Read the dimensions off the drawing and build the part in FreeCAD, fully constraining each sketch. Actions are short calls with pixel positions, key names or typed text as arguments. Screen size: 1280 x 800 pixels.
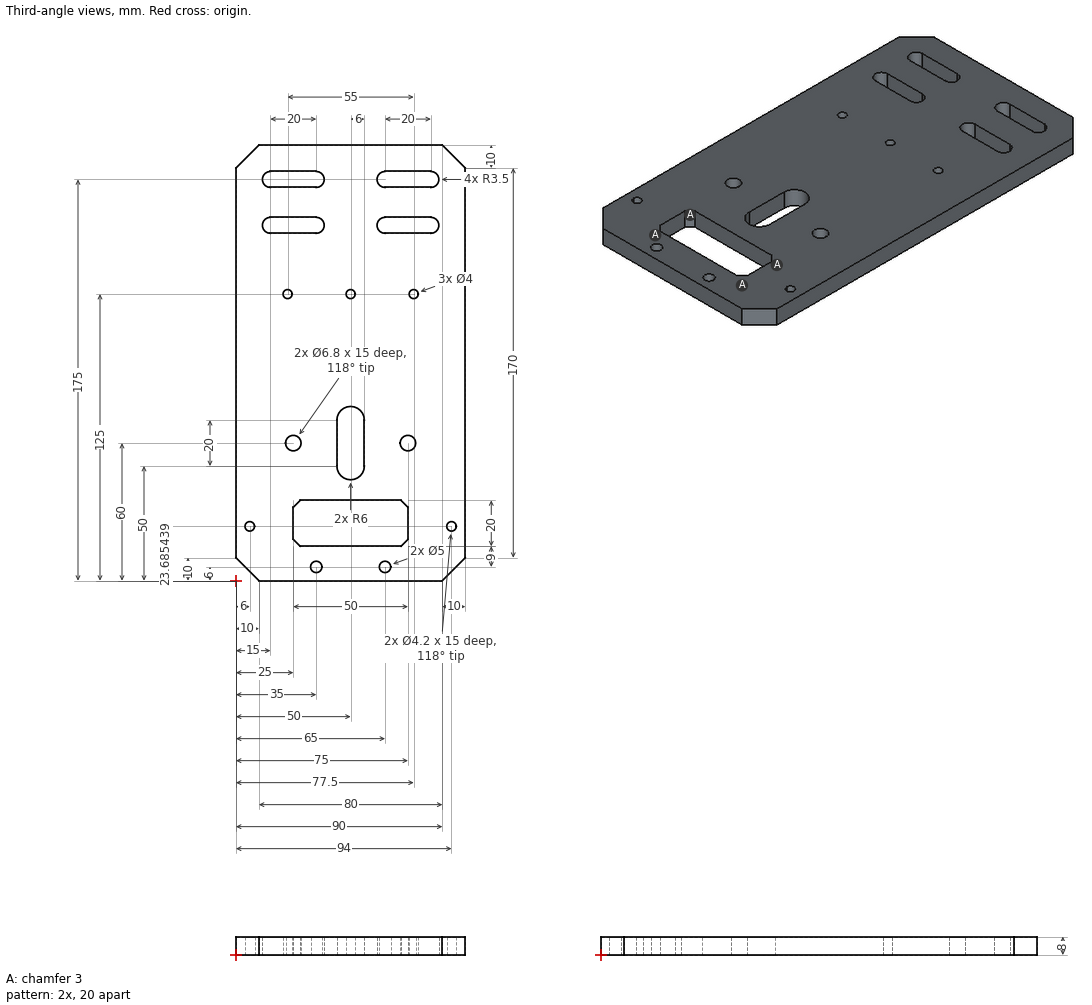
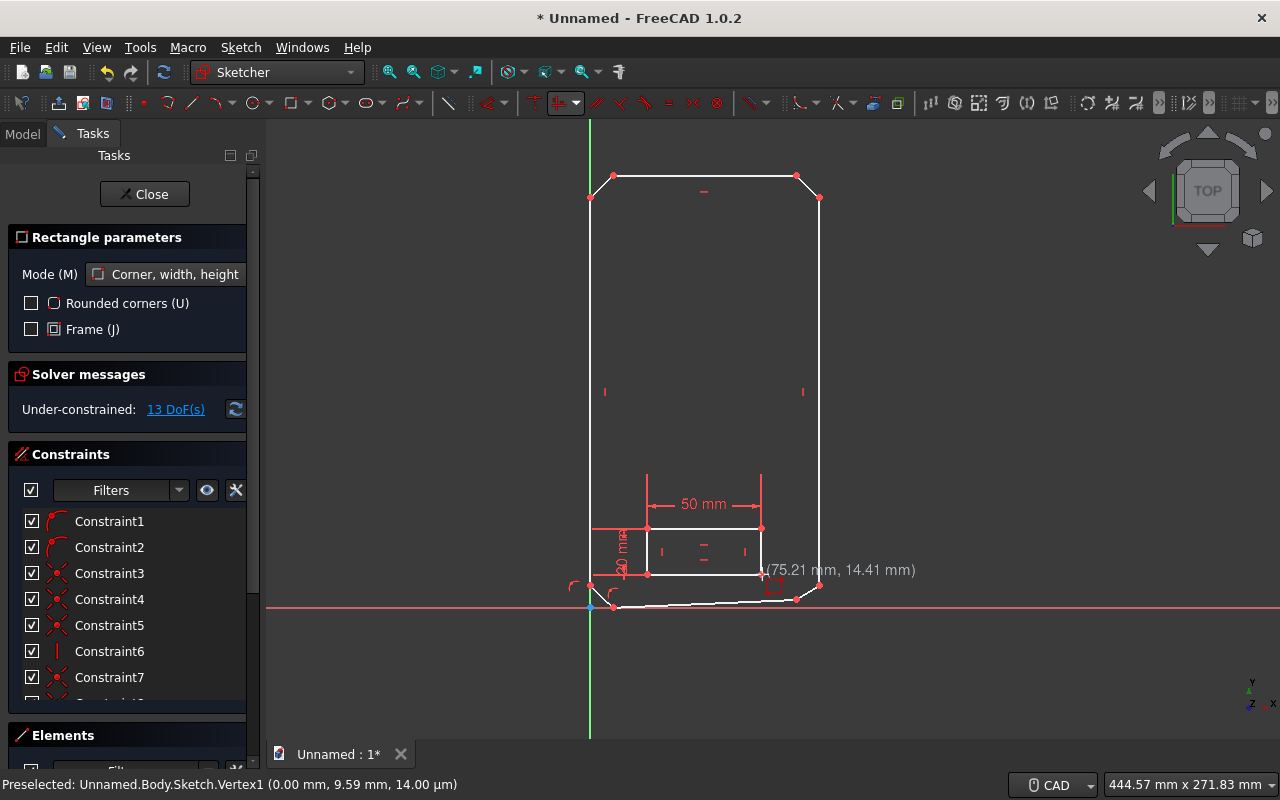
click(366, 104)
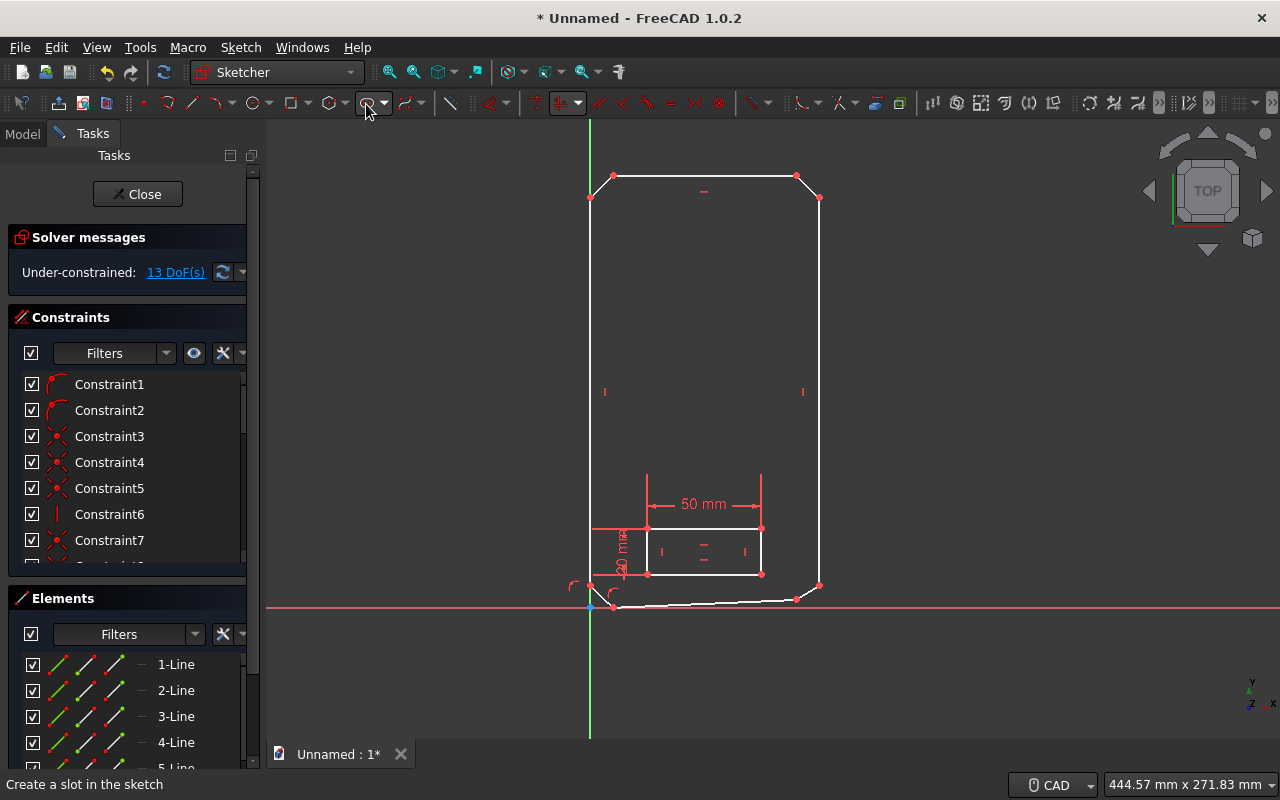
scroll(704, 494, up, 3)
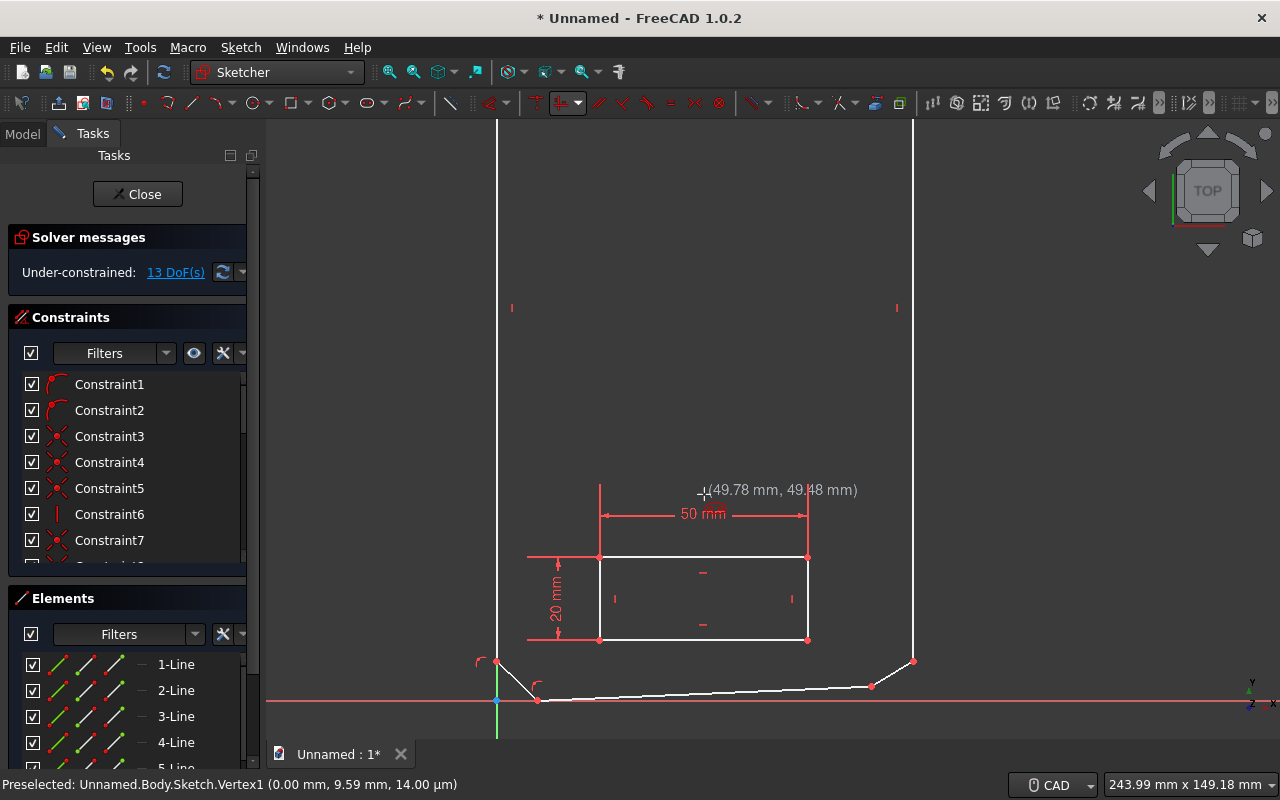
click(705, 493)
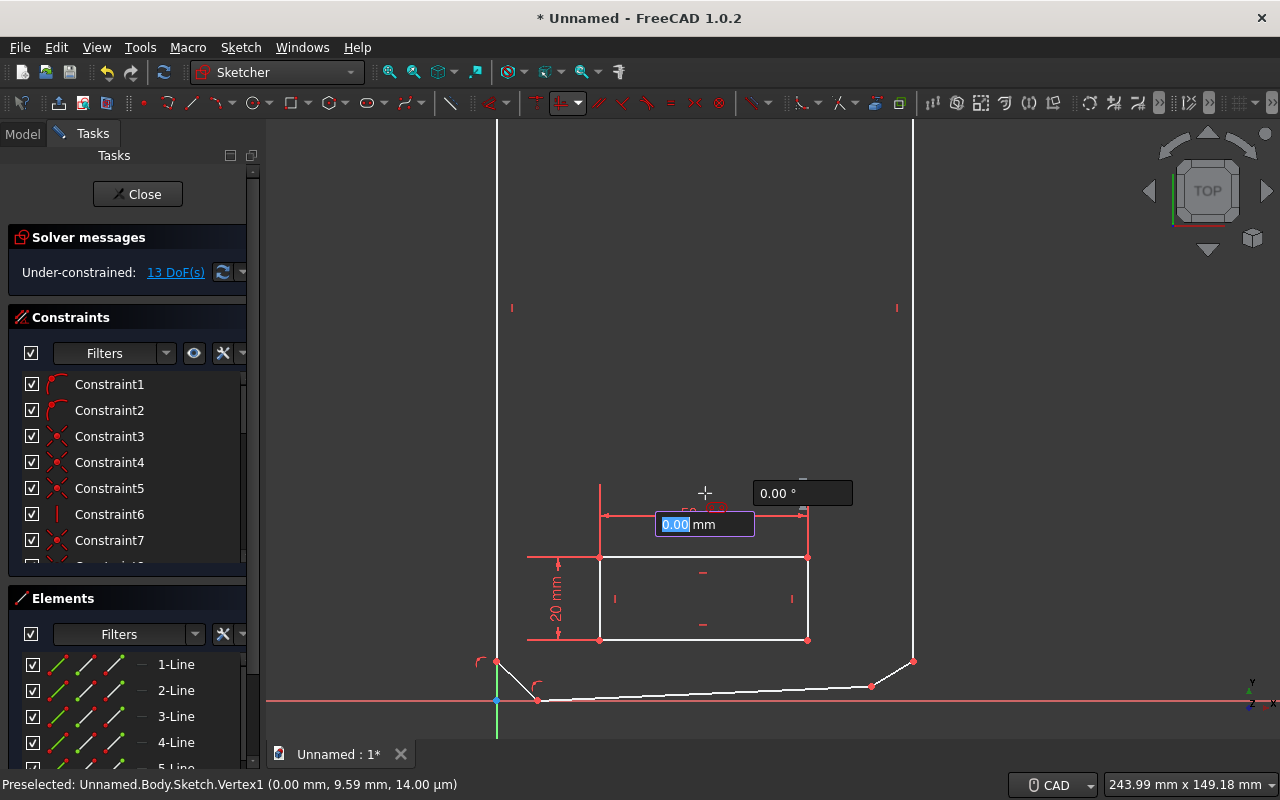
click(705, 410)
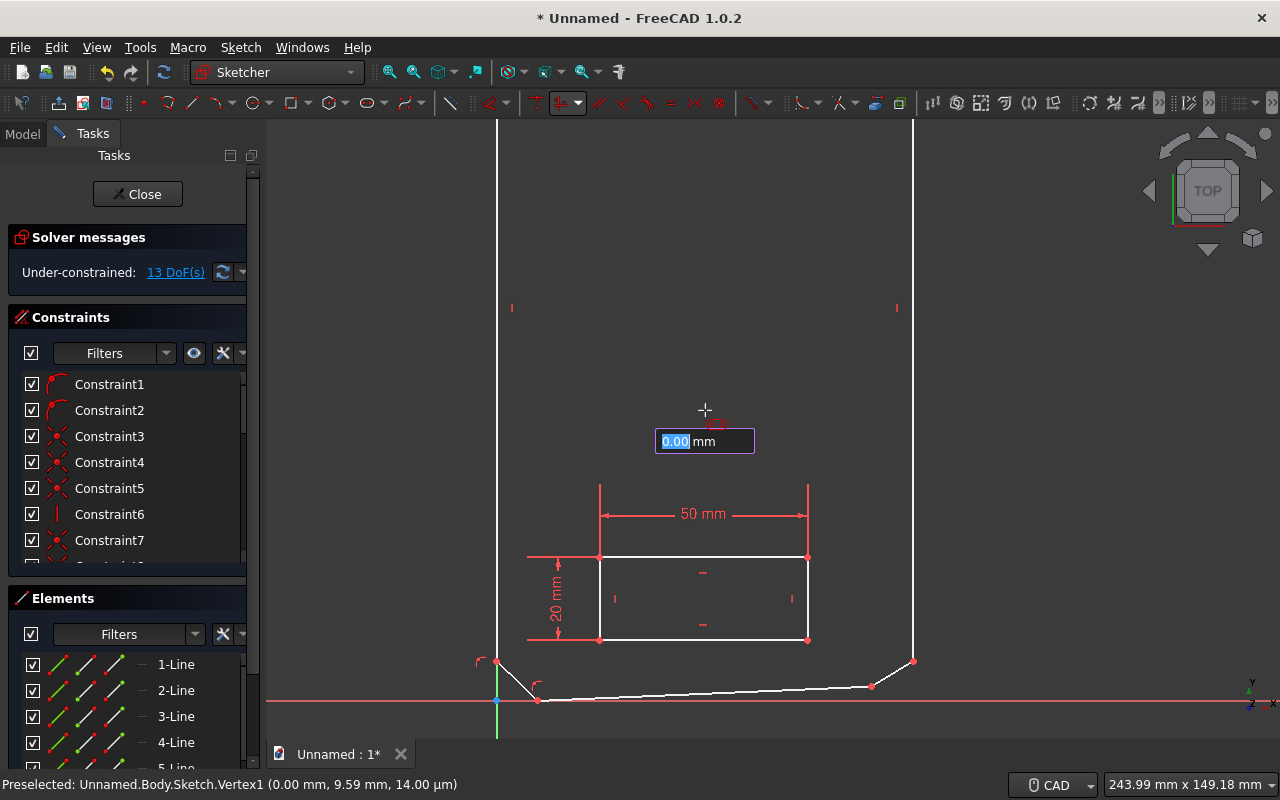
click(729, 452)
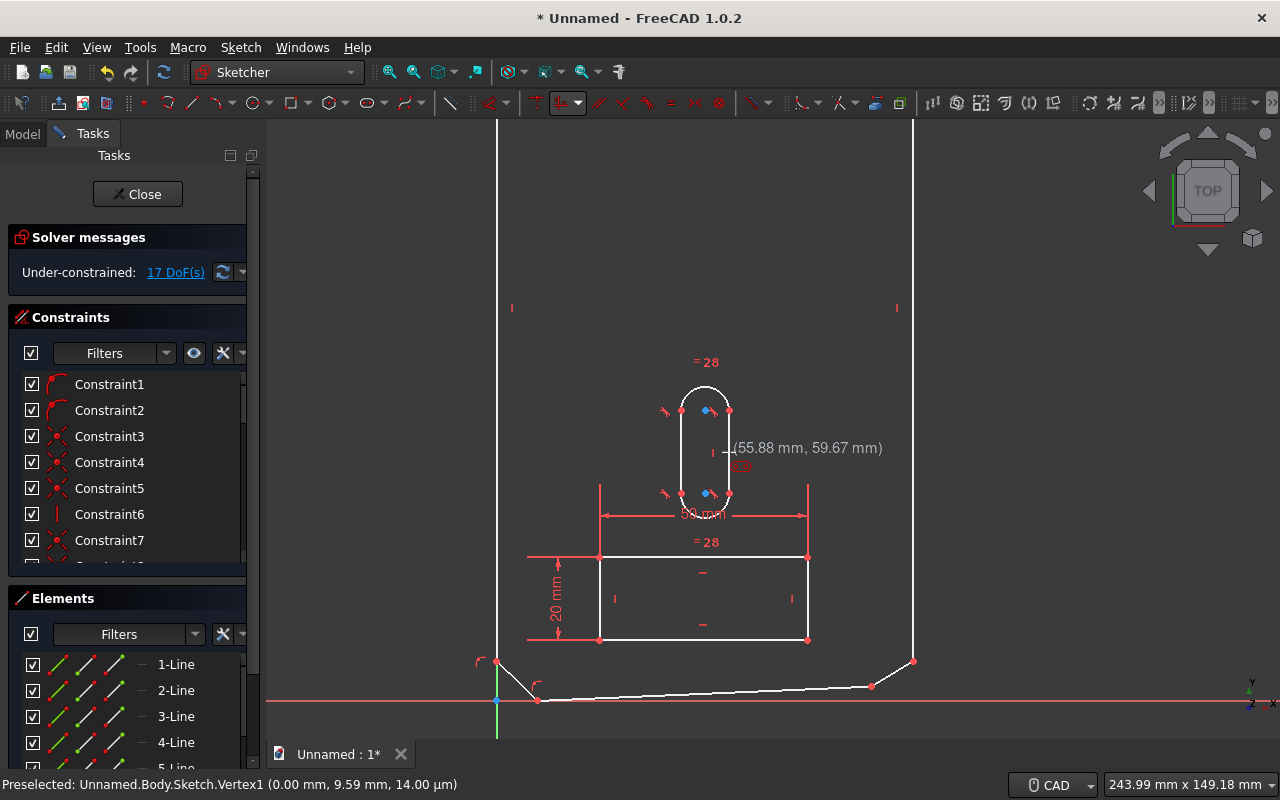
click(254, 104)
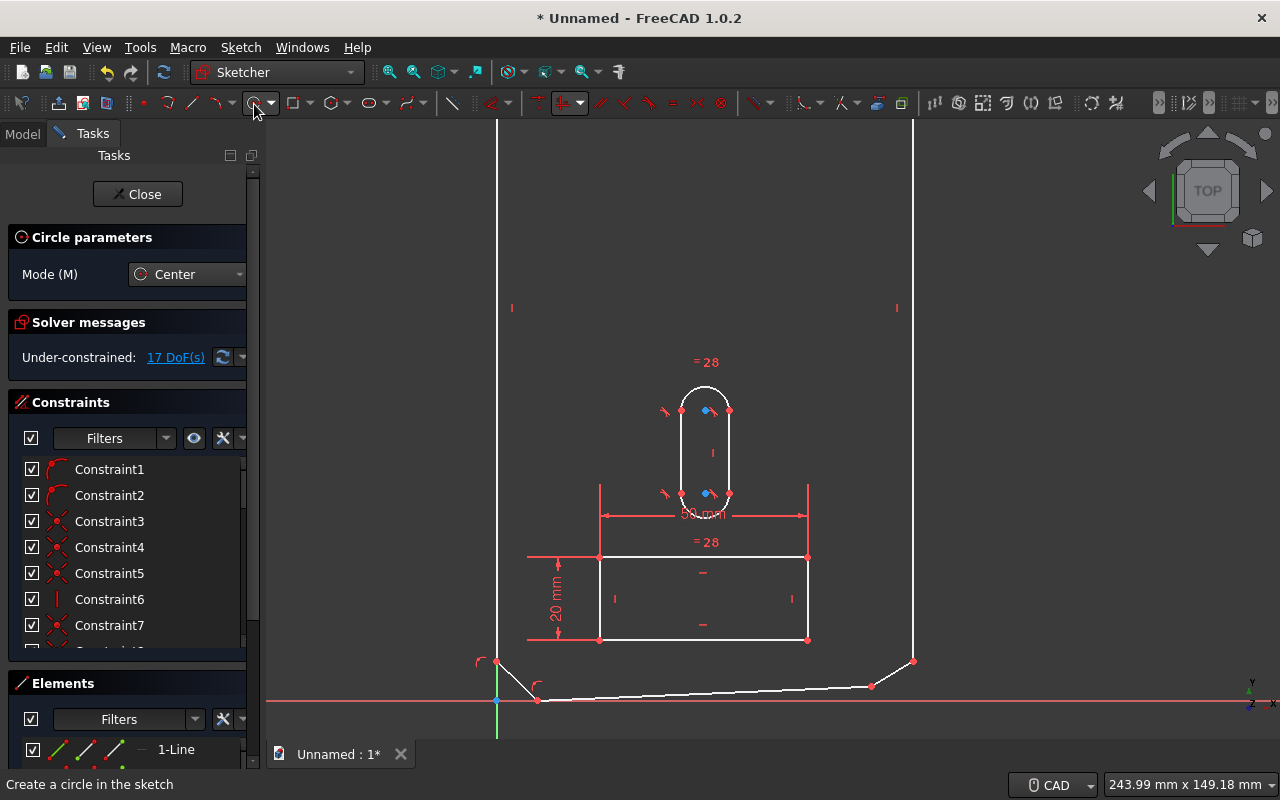
scroll(767, 676, up, 4)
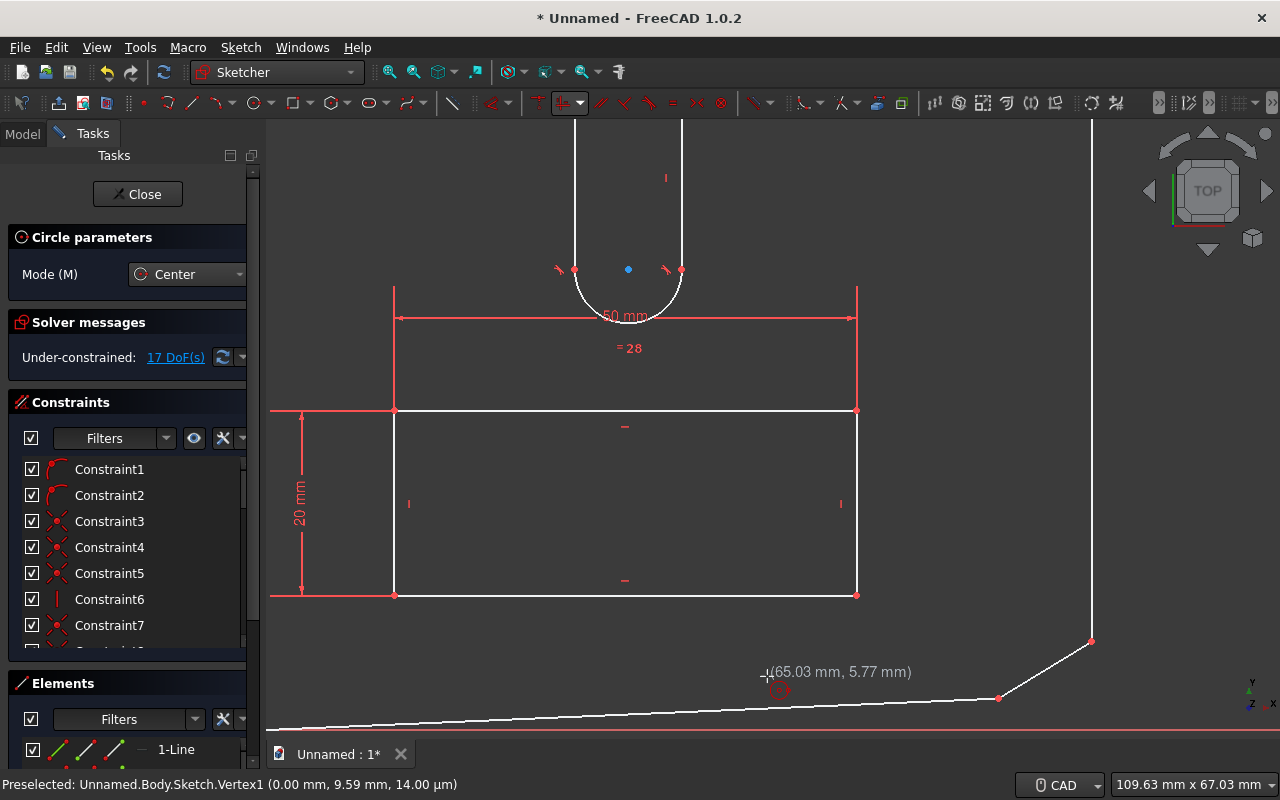
scroll(730, 618, down, 7)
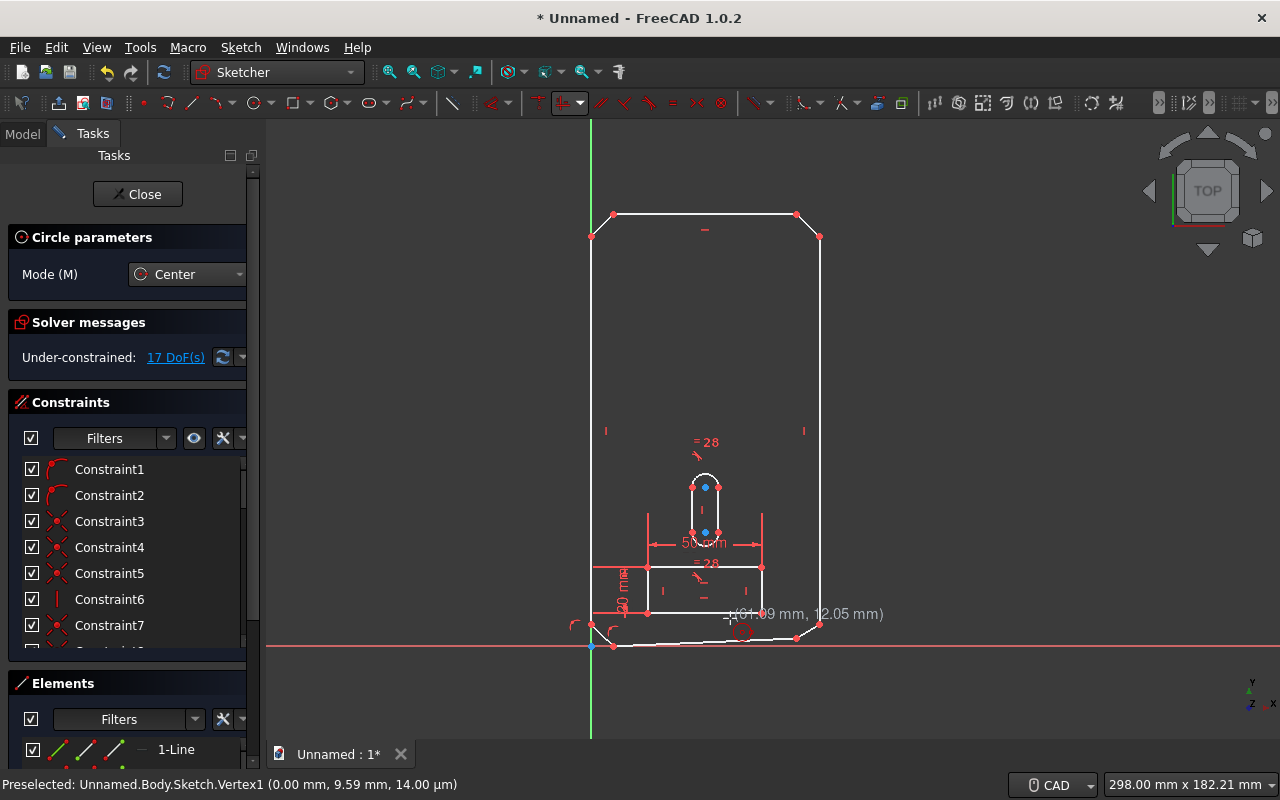
click(739, 633)
move(743, 629)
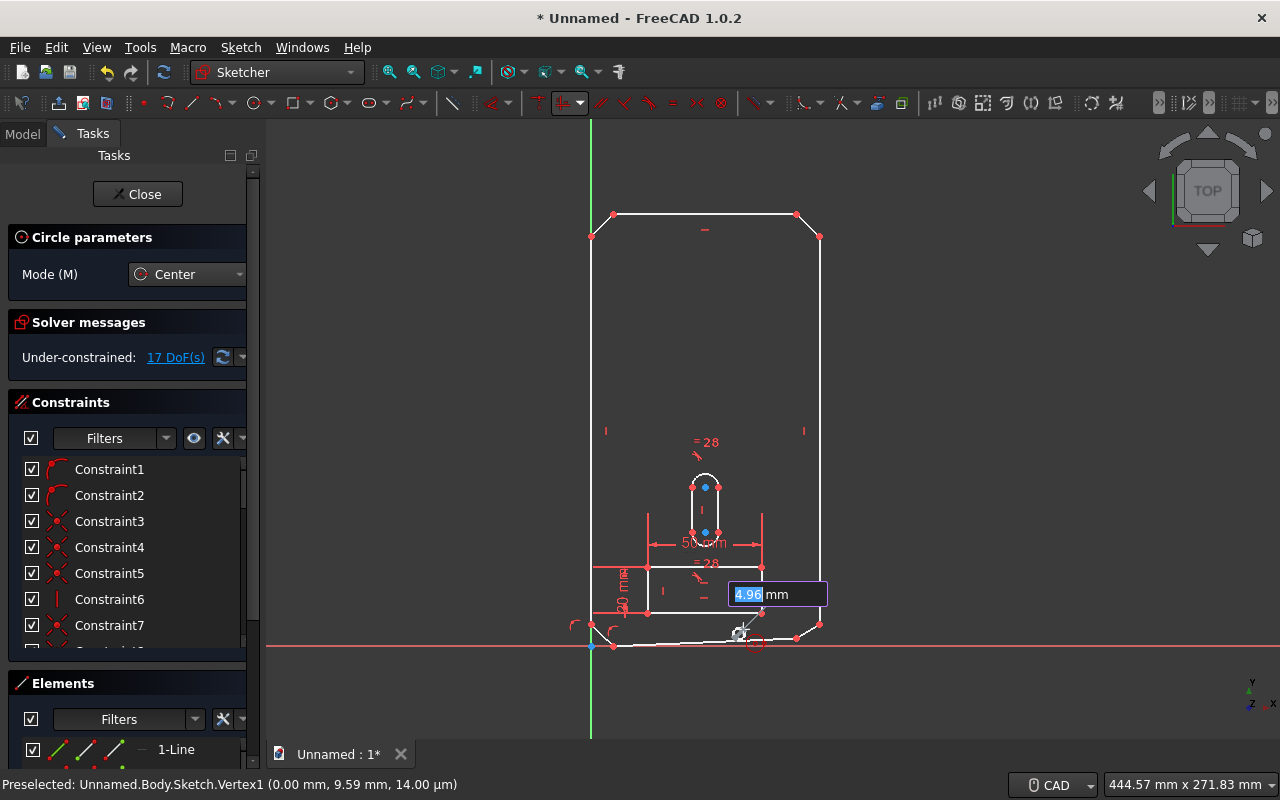
text(5)
key(Return)